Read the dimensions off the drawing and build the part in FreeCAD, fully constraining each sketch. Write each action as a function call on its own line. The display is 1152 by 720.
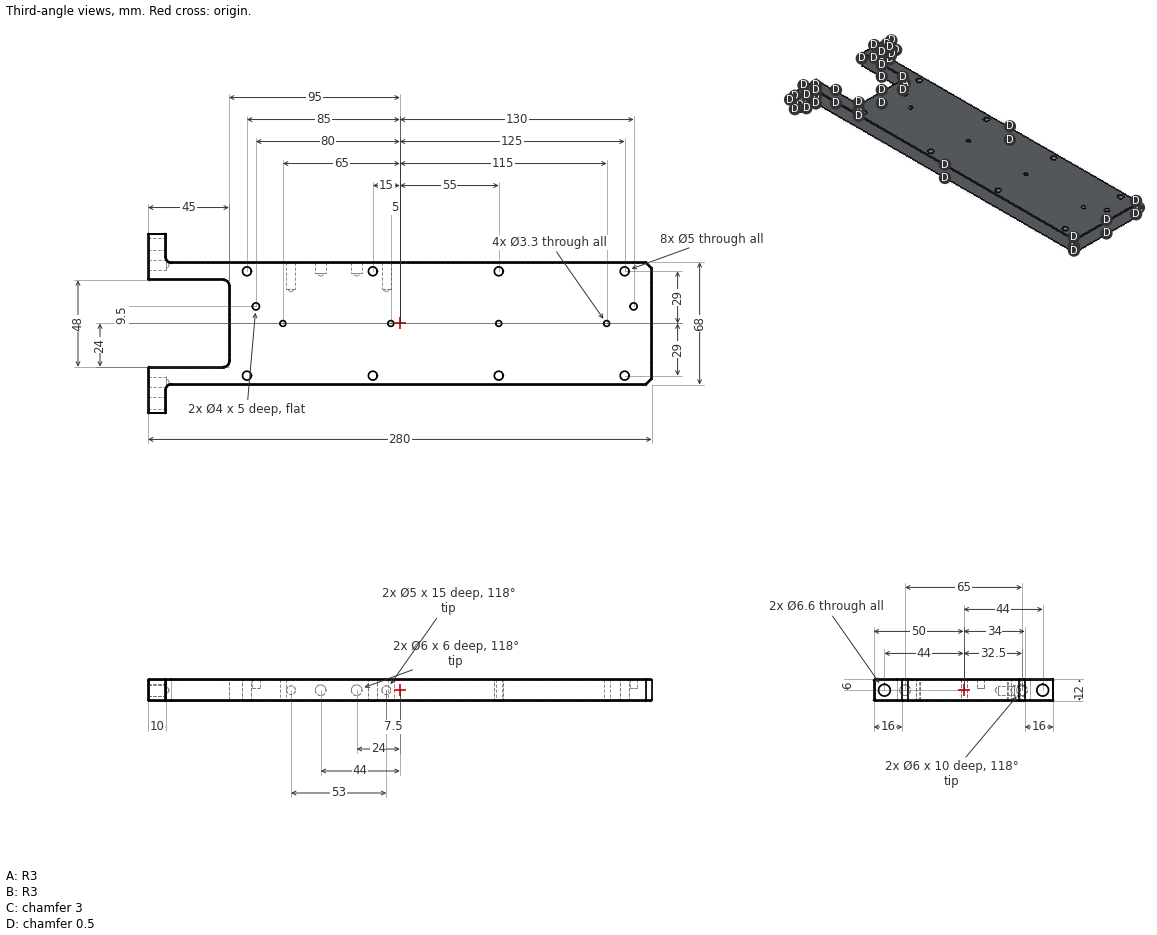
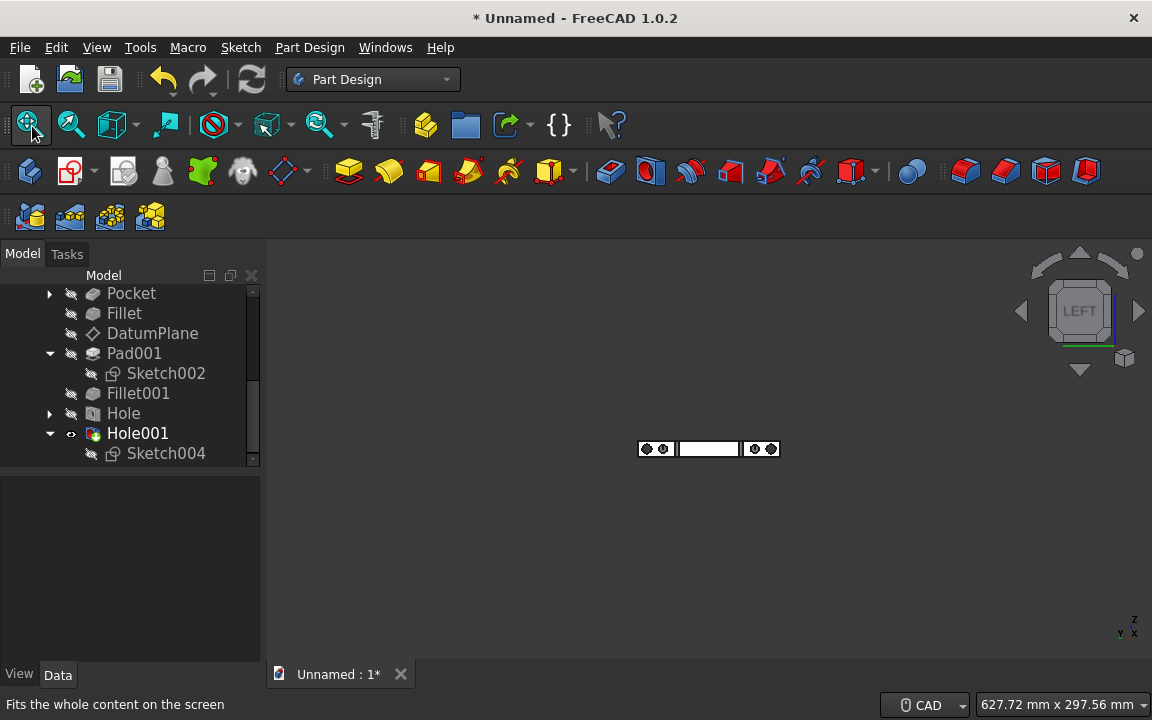
scroll(757, 448, up, 5)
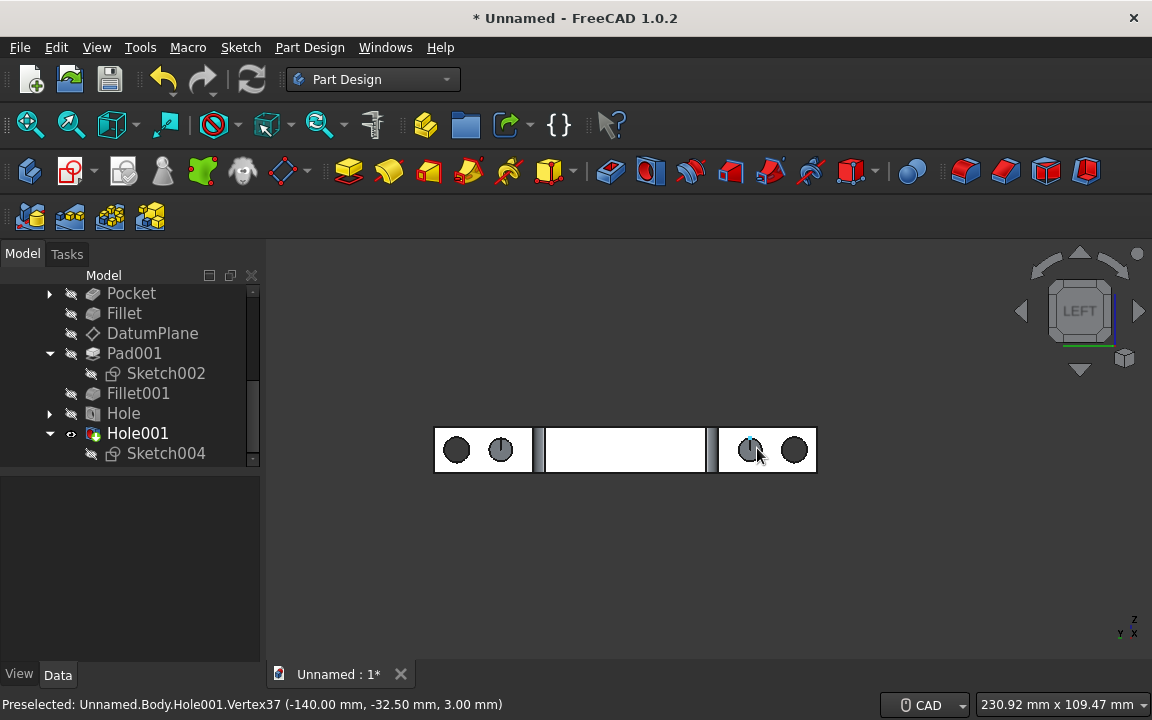
click(32, 126)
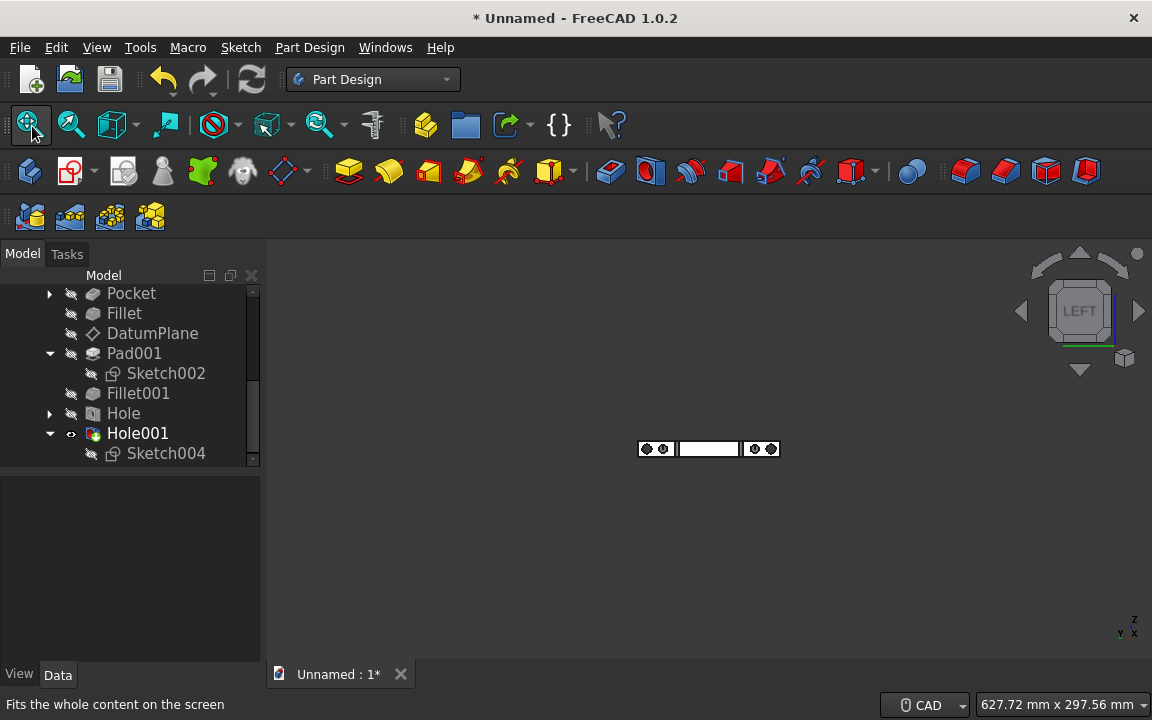
key(0)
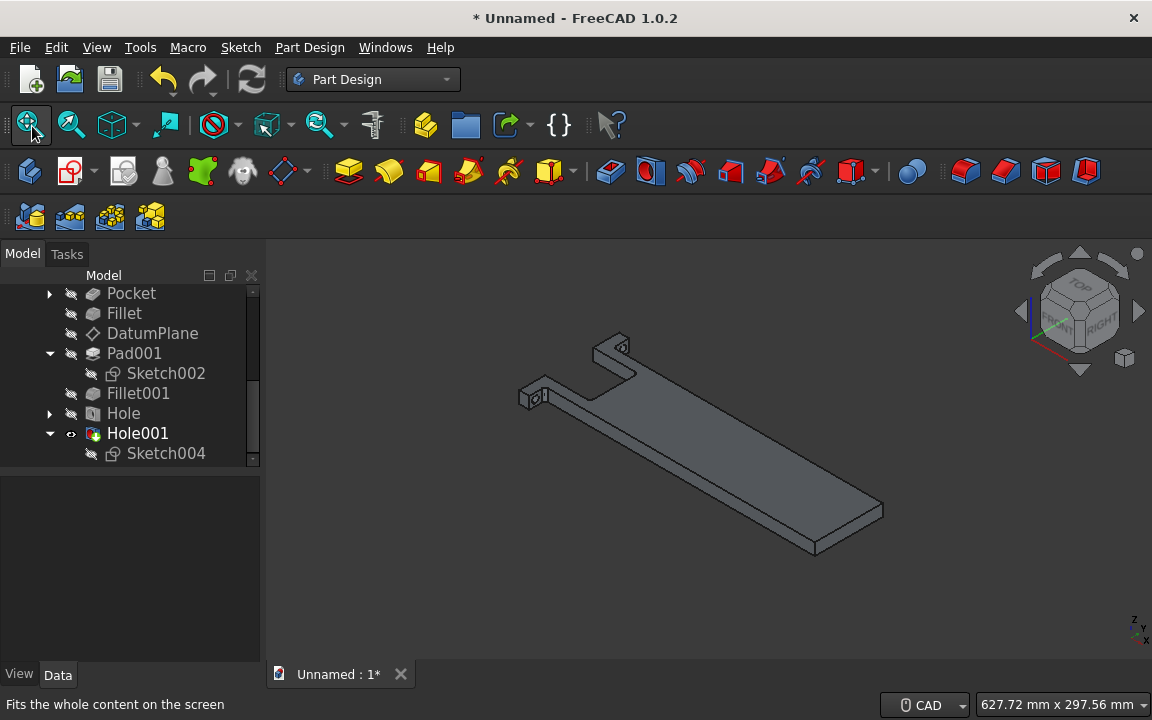
click(815, 548)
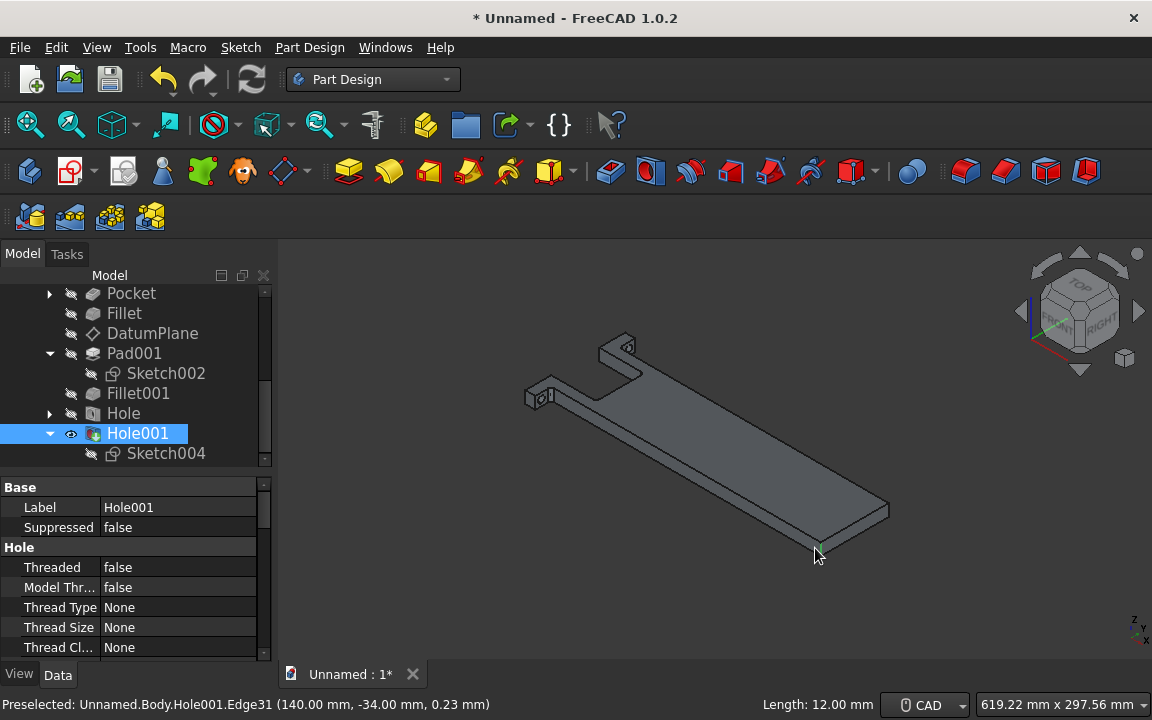
scroll(889, 509, up, 5)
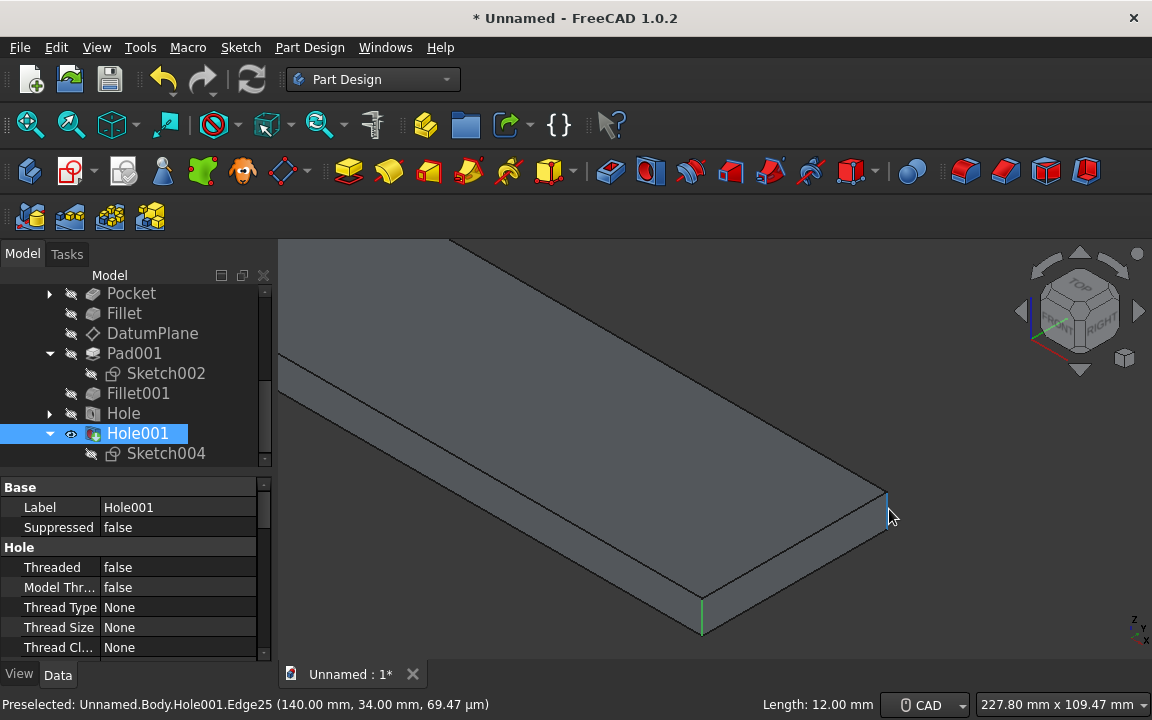
click(32, 126)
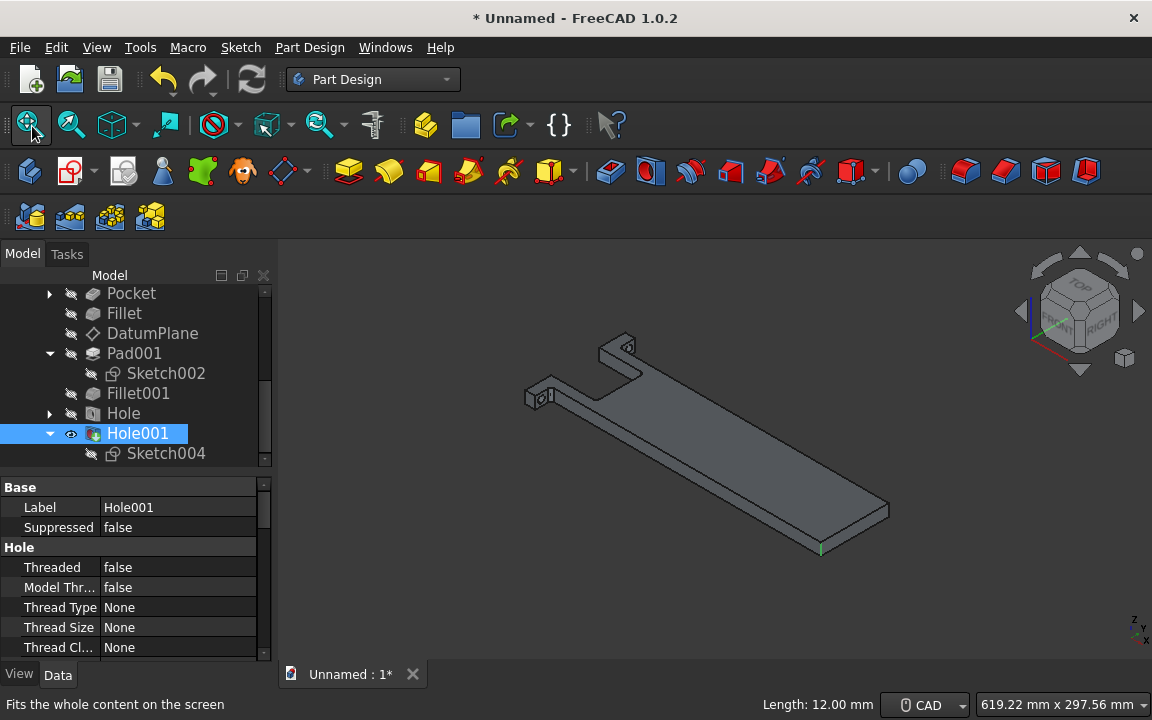
key(2)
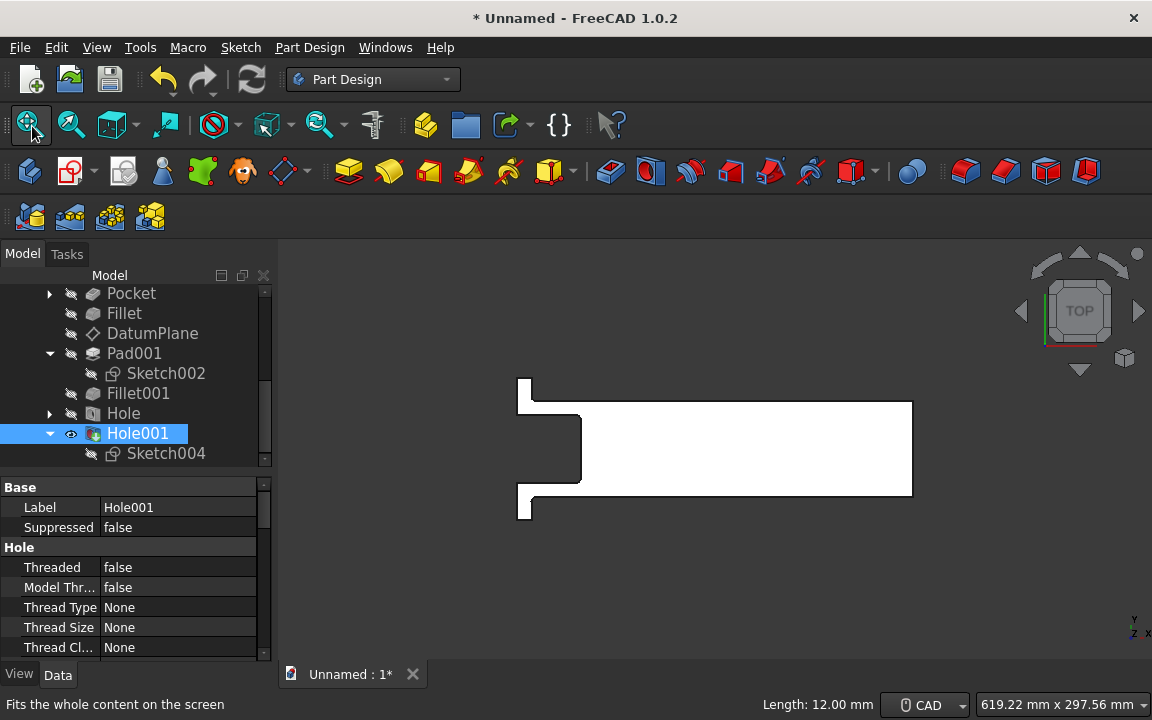
scroll(913, 400, up, 5)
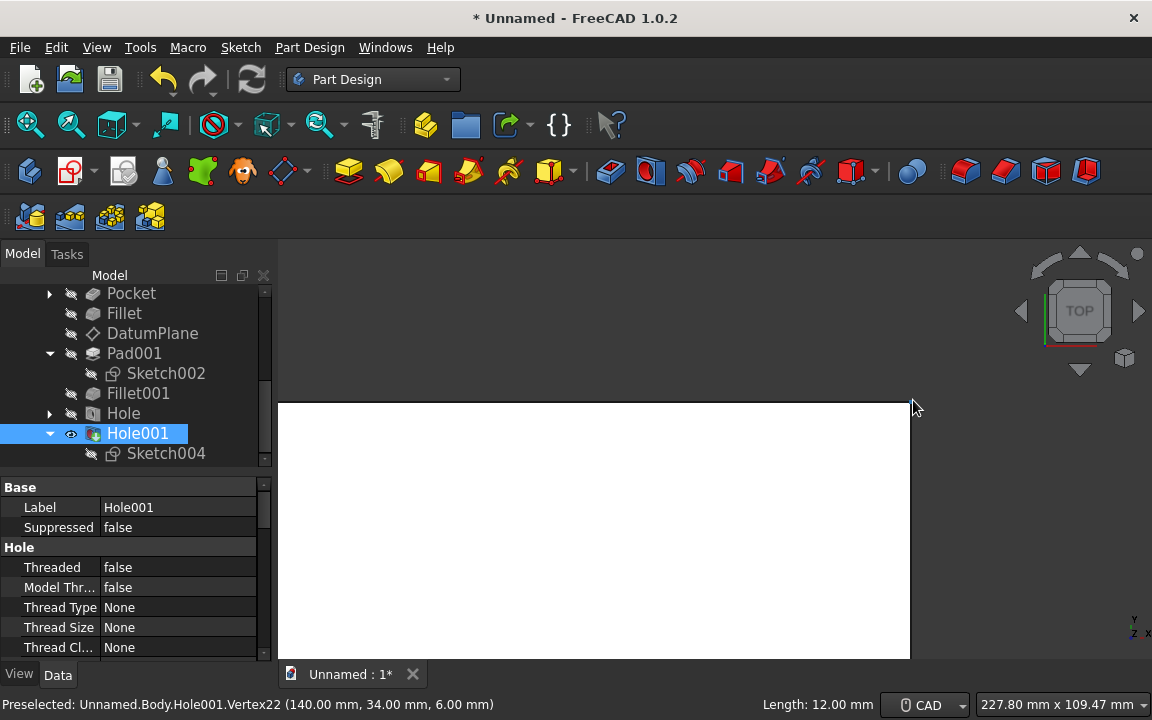
click(32, 126)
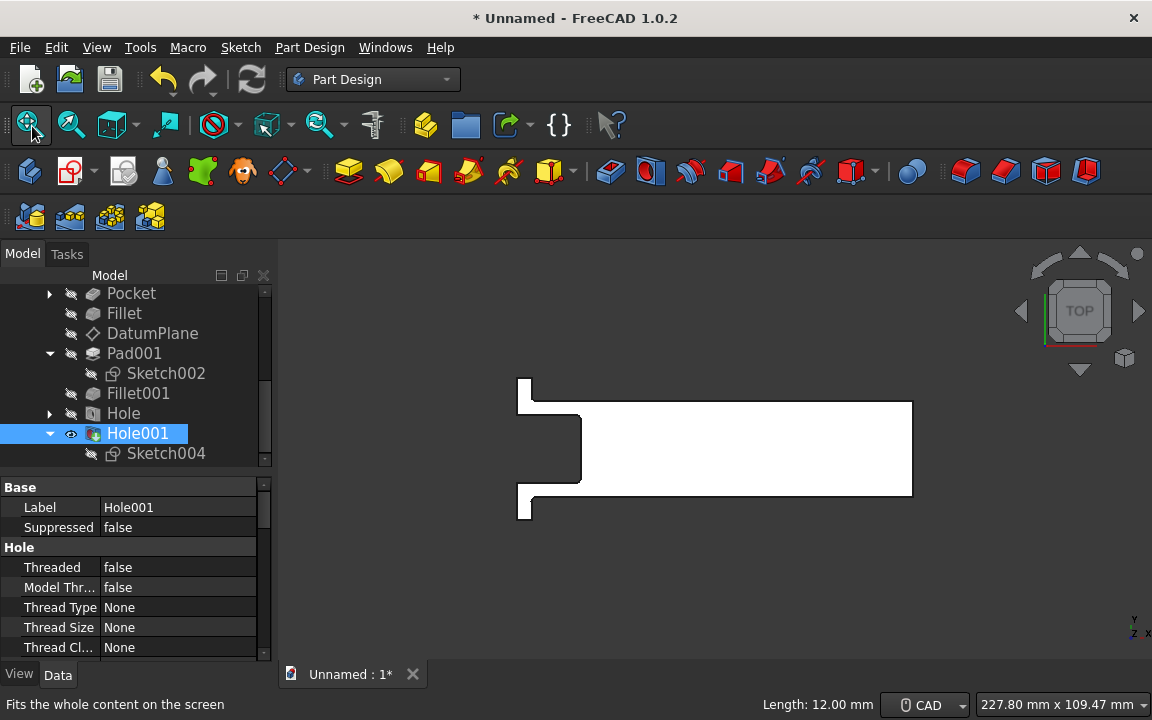
key(1)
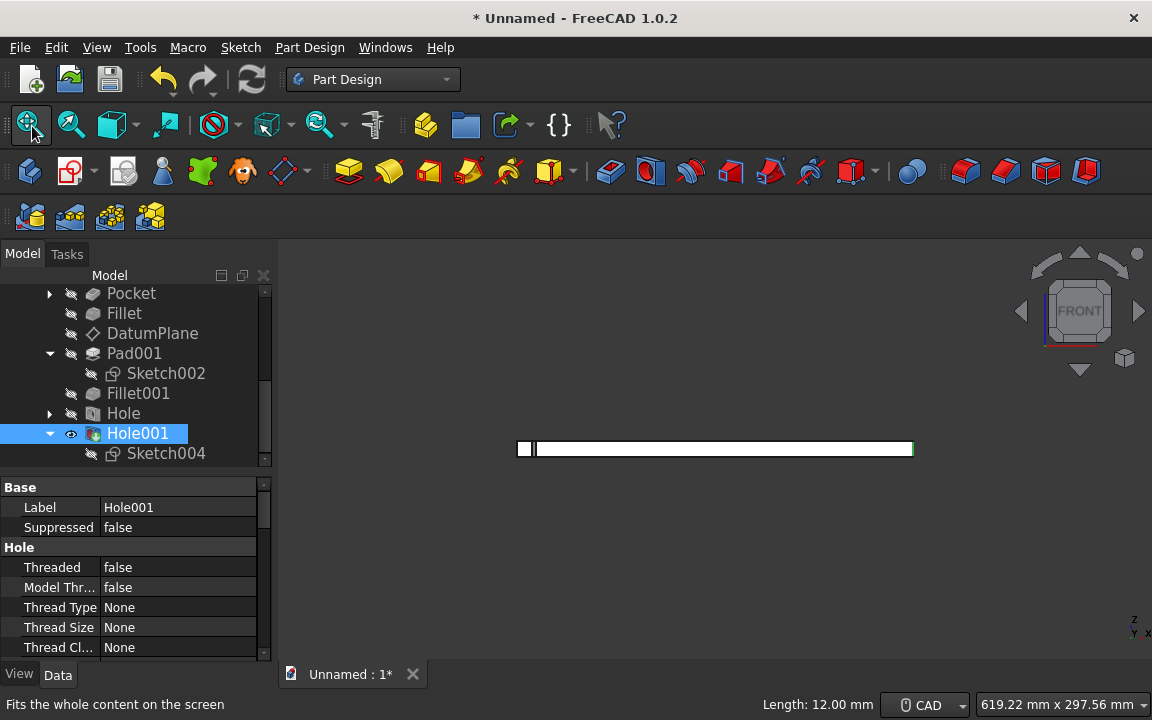
scroll(913, 448, up, 5)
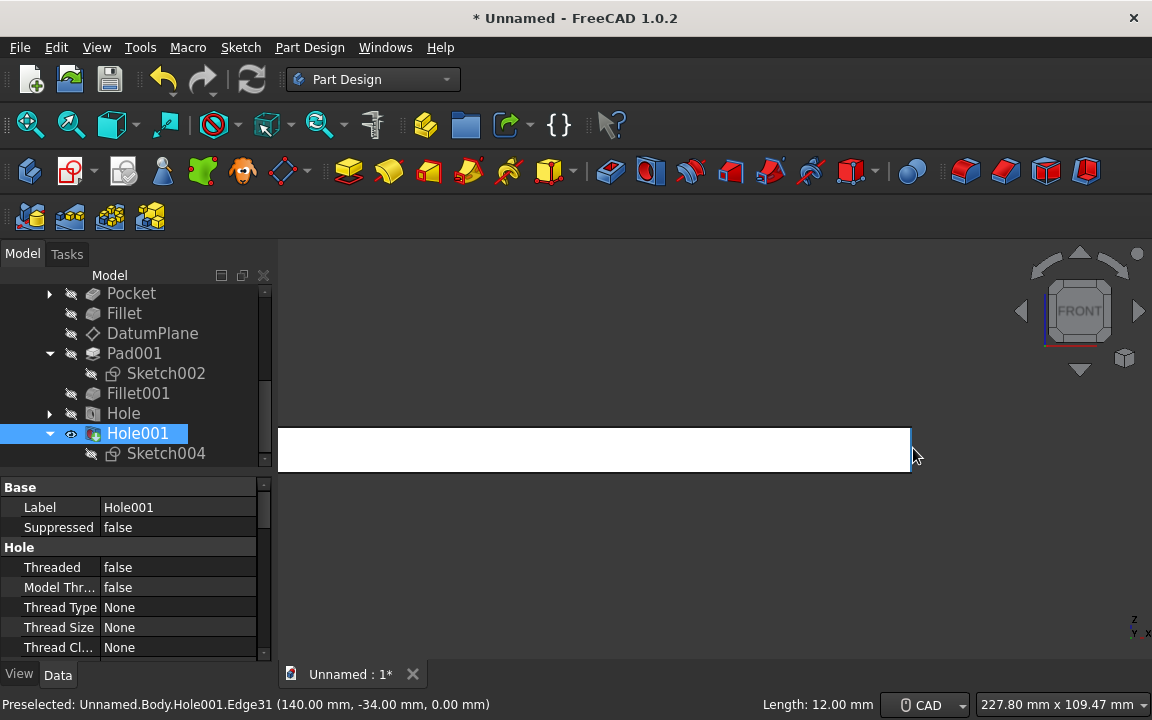
click(32, 126)